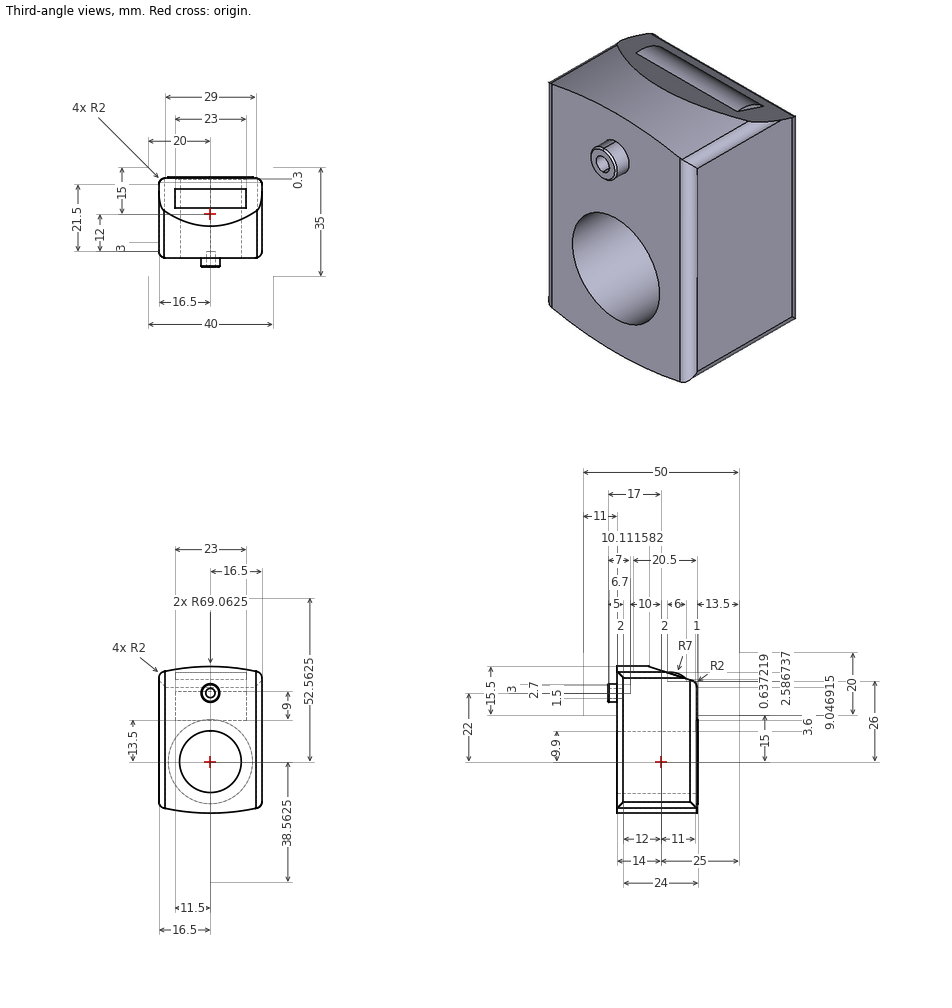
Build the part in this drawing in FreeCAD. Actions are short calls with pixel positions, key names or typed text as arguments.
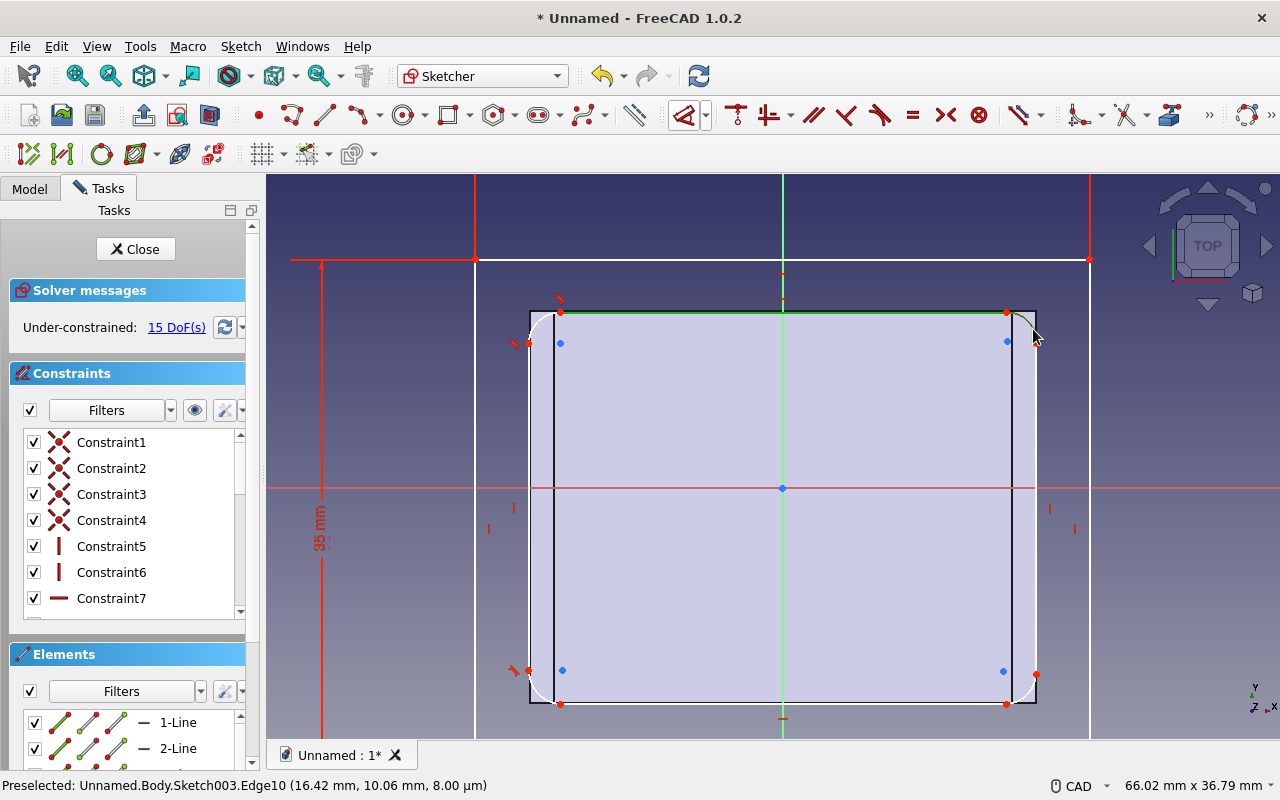
click(880, 116)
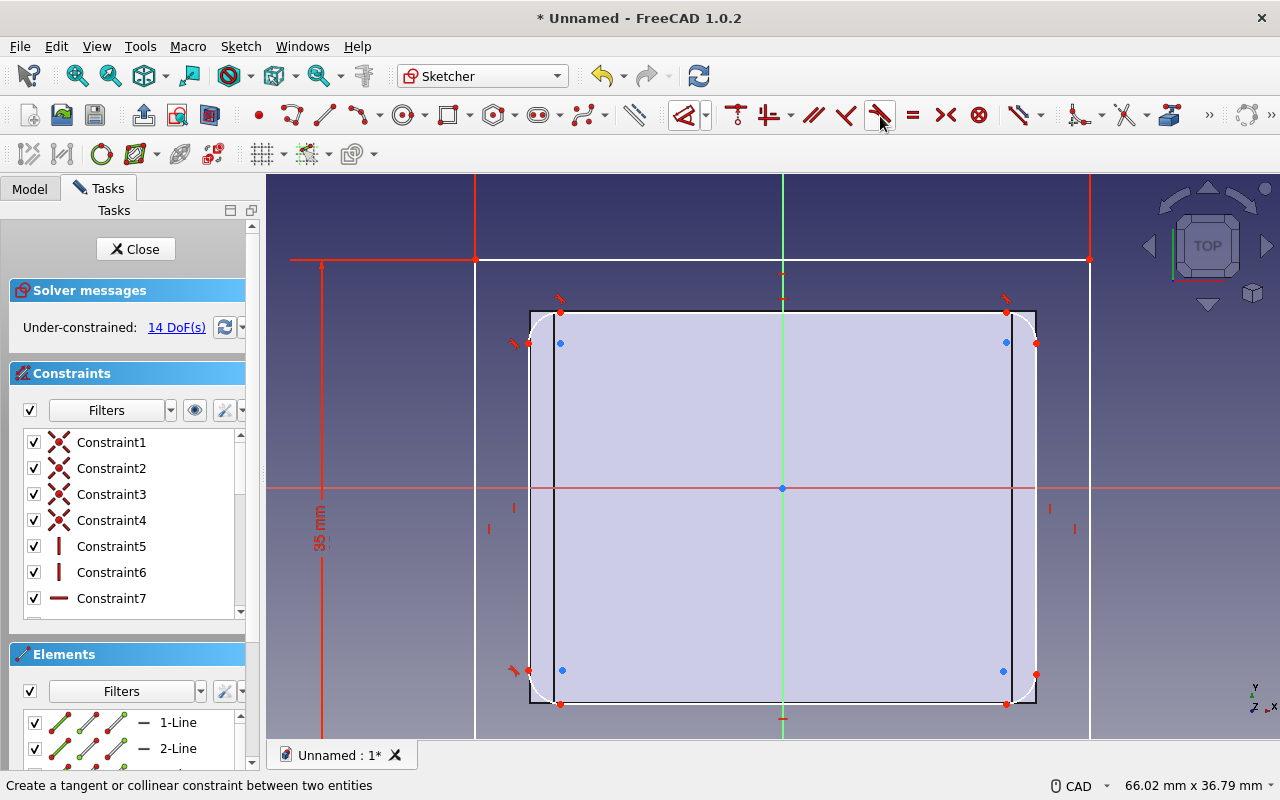
click(1036, 442)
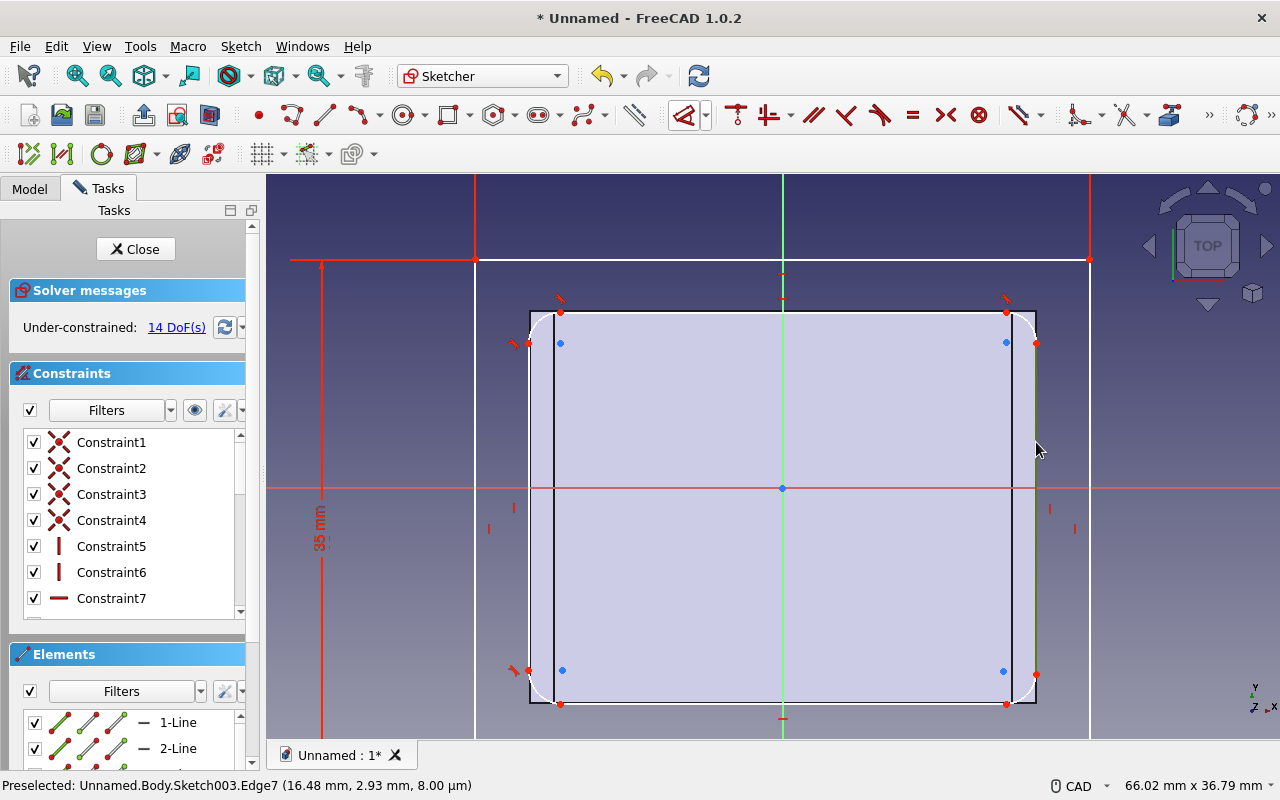
click(1033, 329)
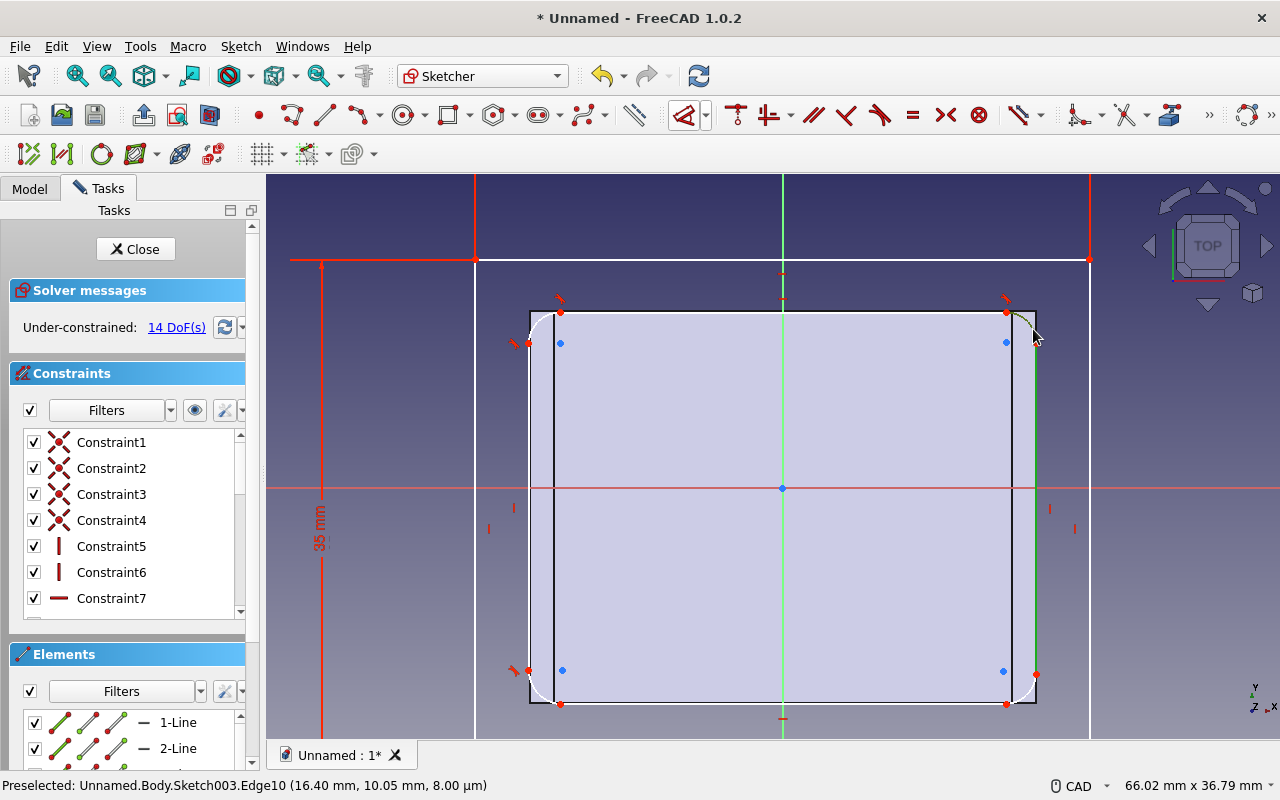
click(880, 116)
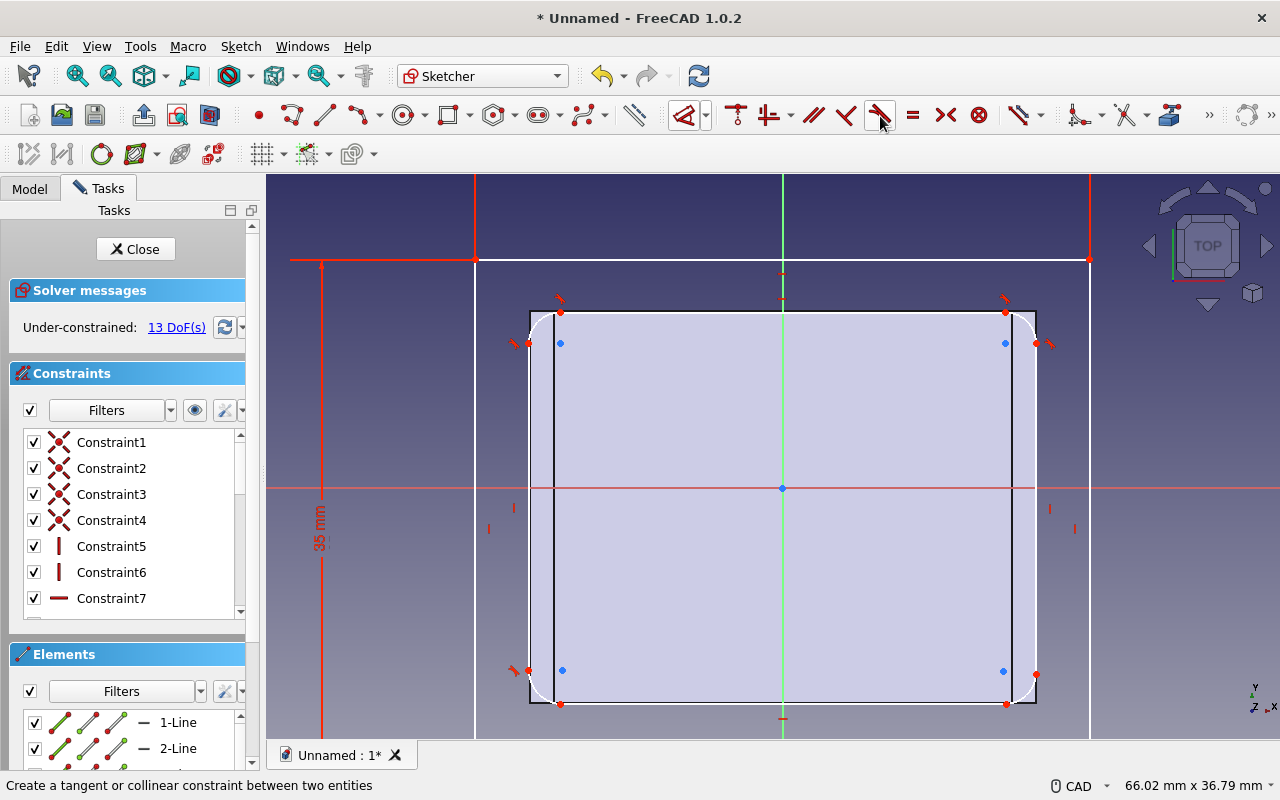
click(1036, 442)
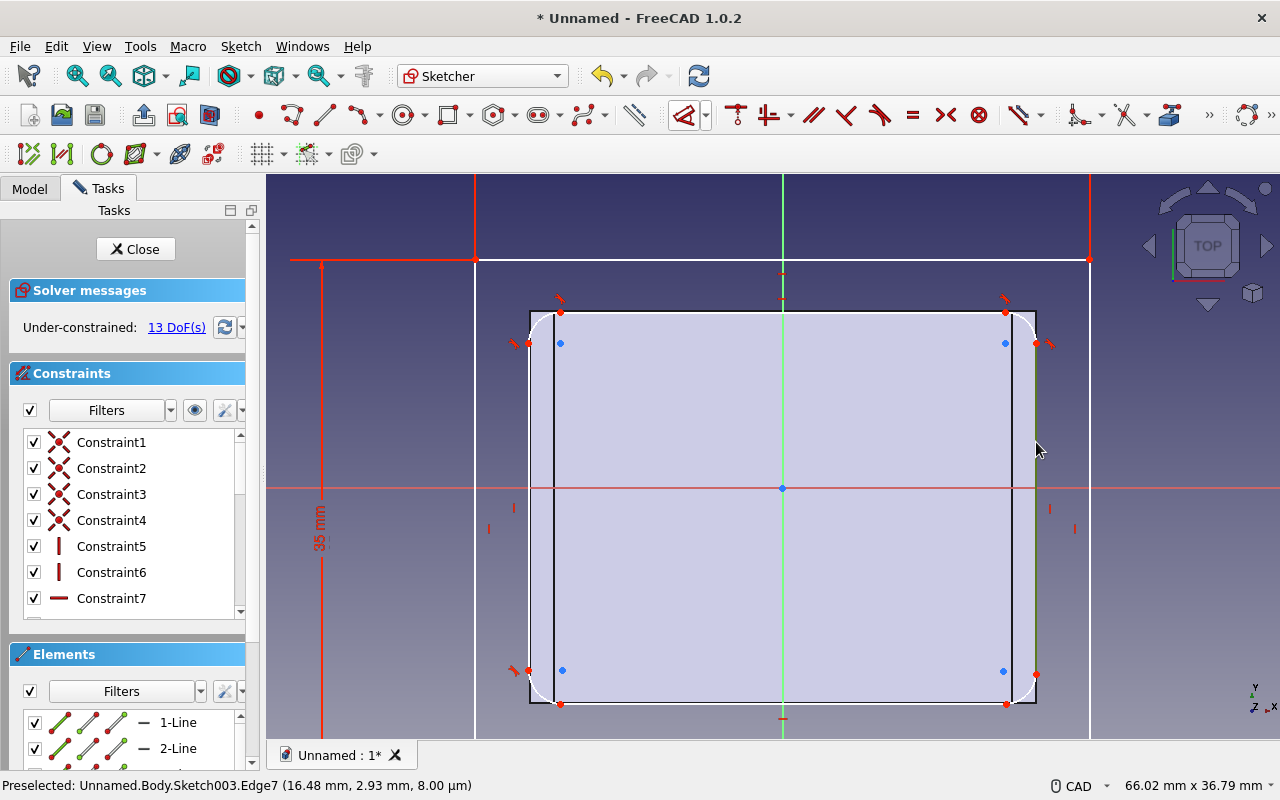
click(1019, 700)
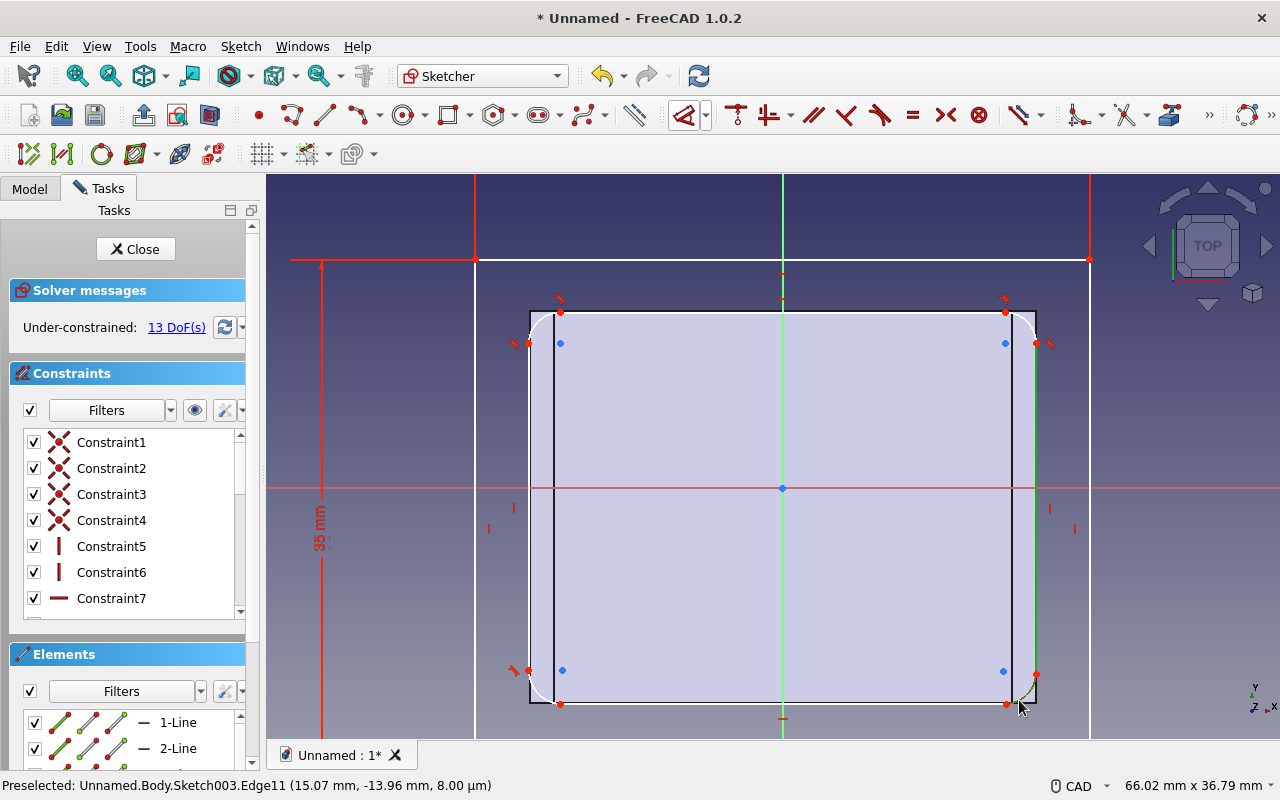
click(880, 116)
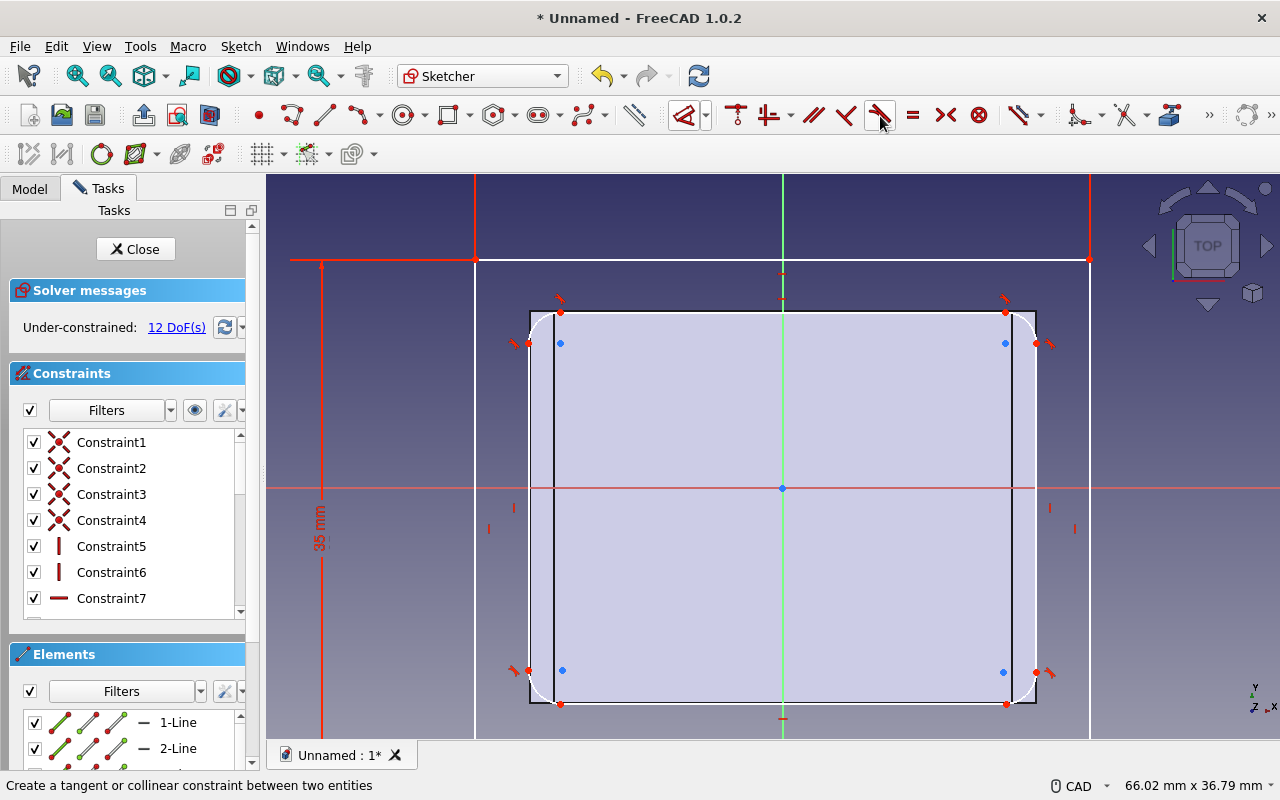
click(872, 704)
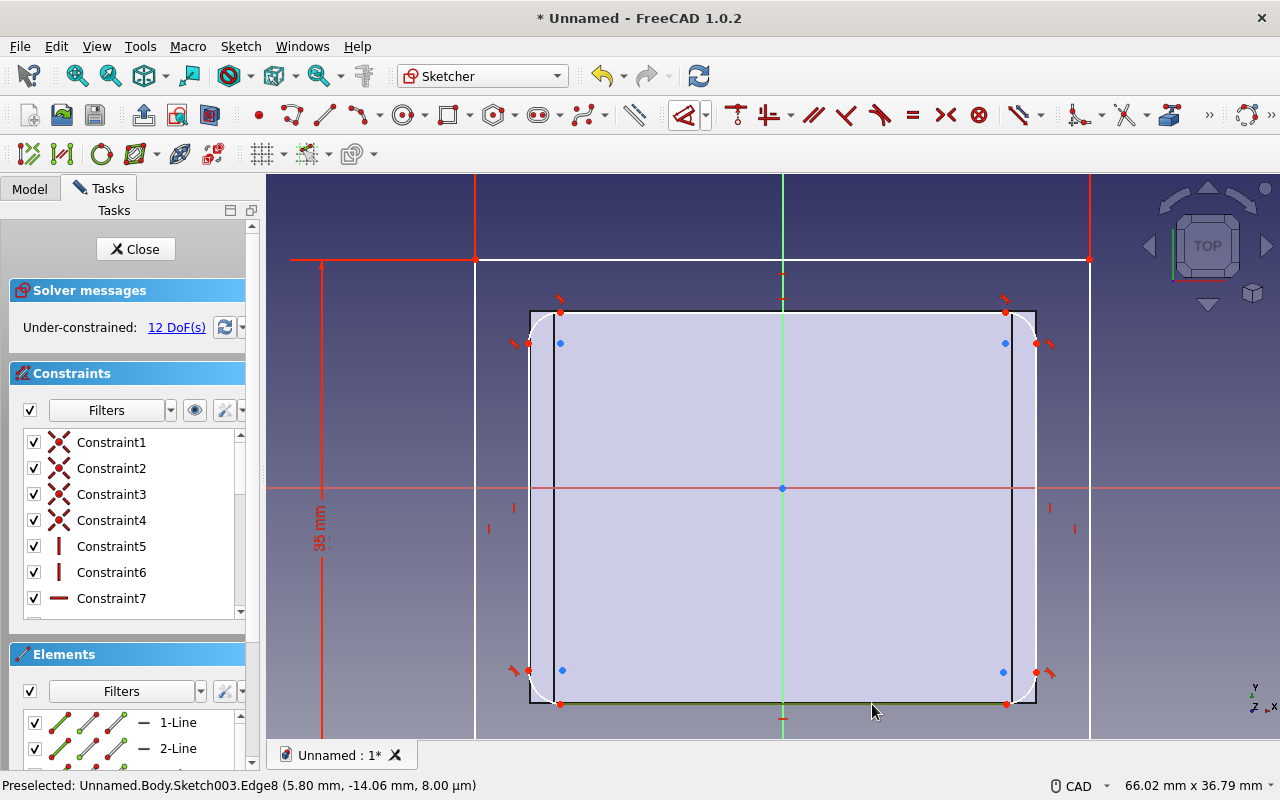
click(1020, 700)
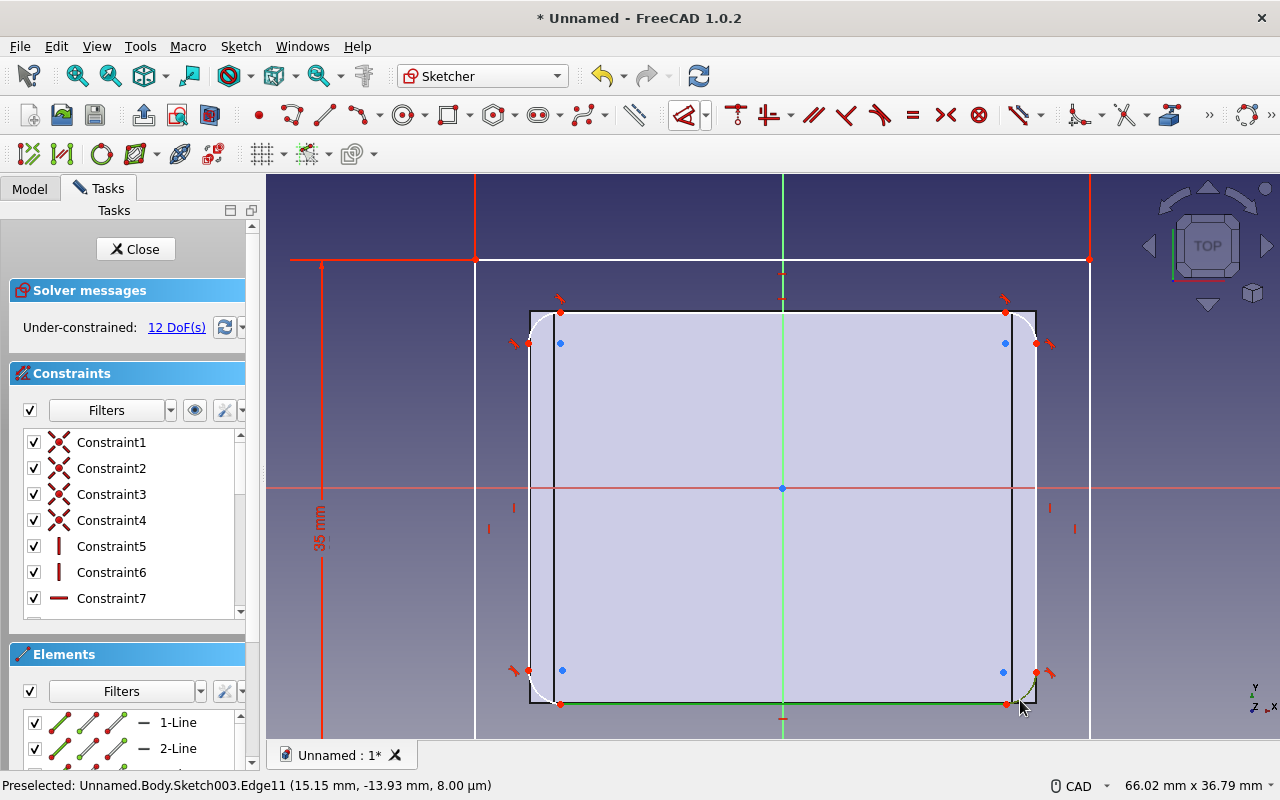
click(880, 116)